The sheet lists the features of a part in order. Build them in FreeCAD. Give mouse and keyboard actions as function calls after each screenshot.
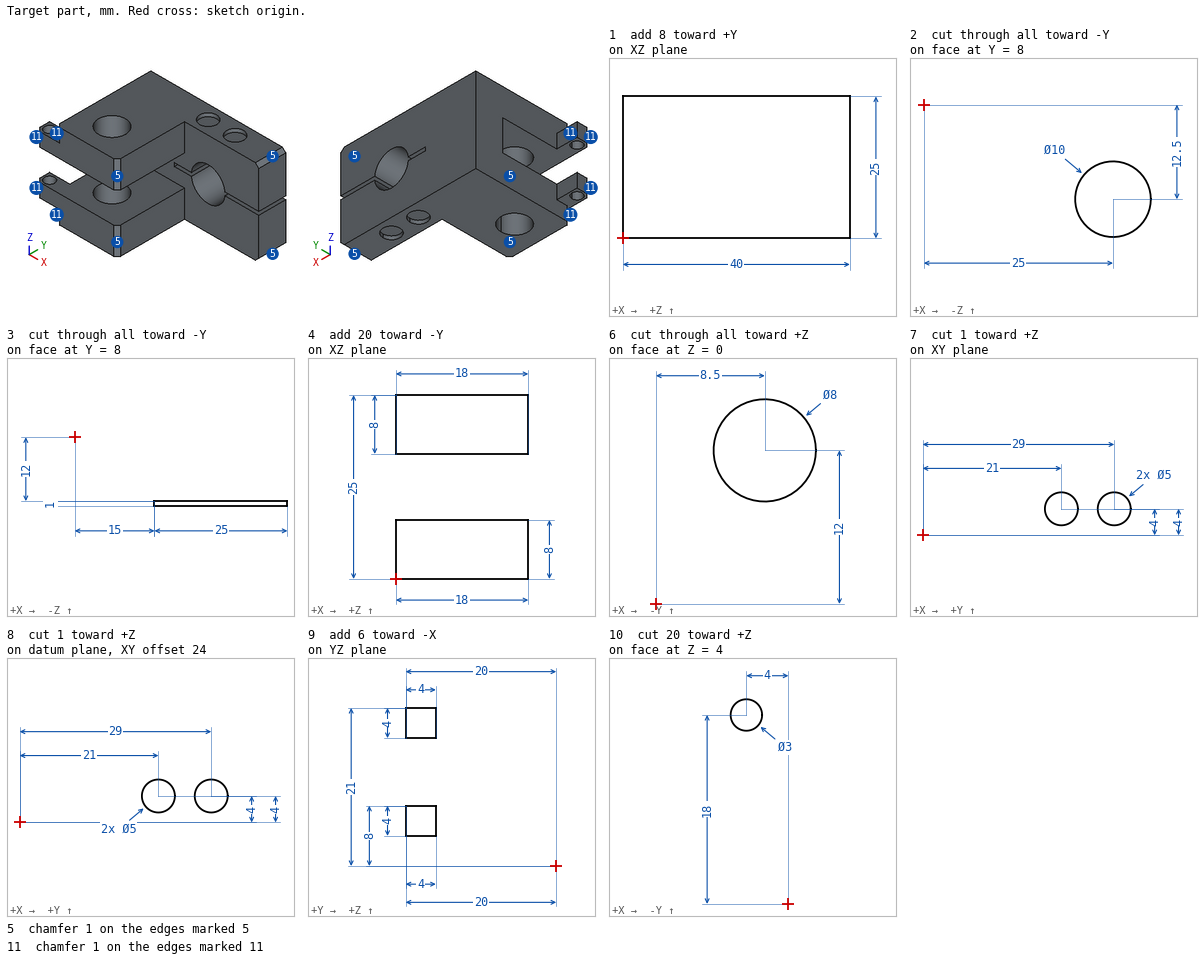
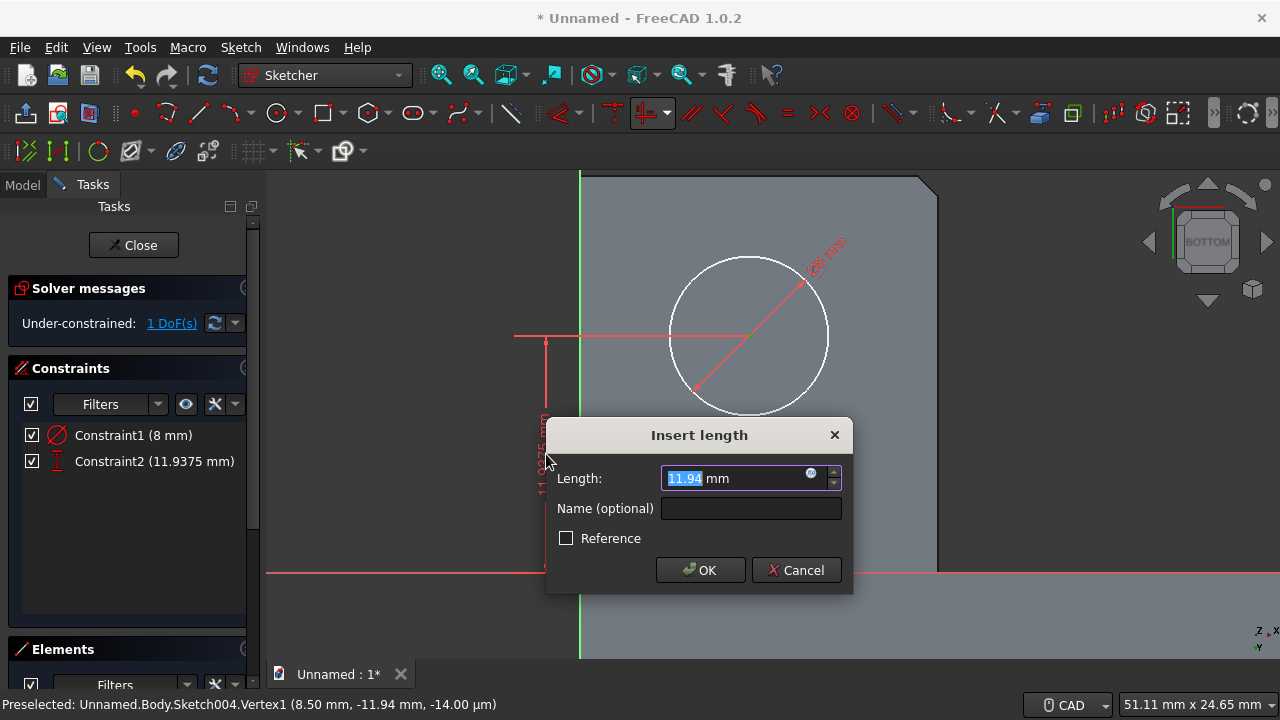
text(12)
key(Return)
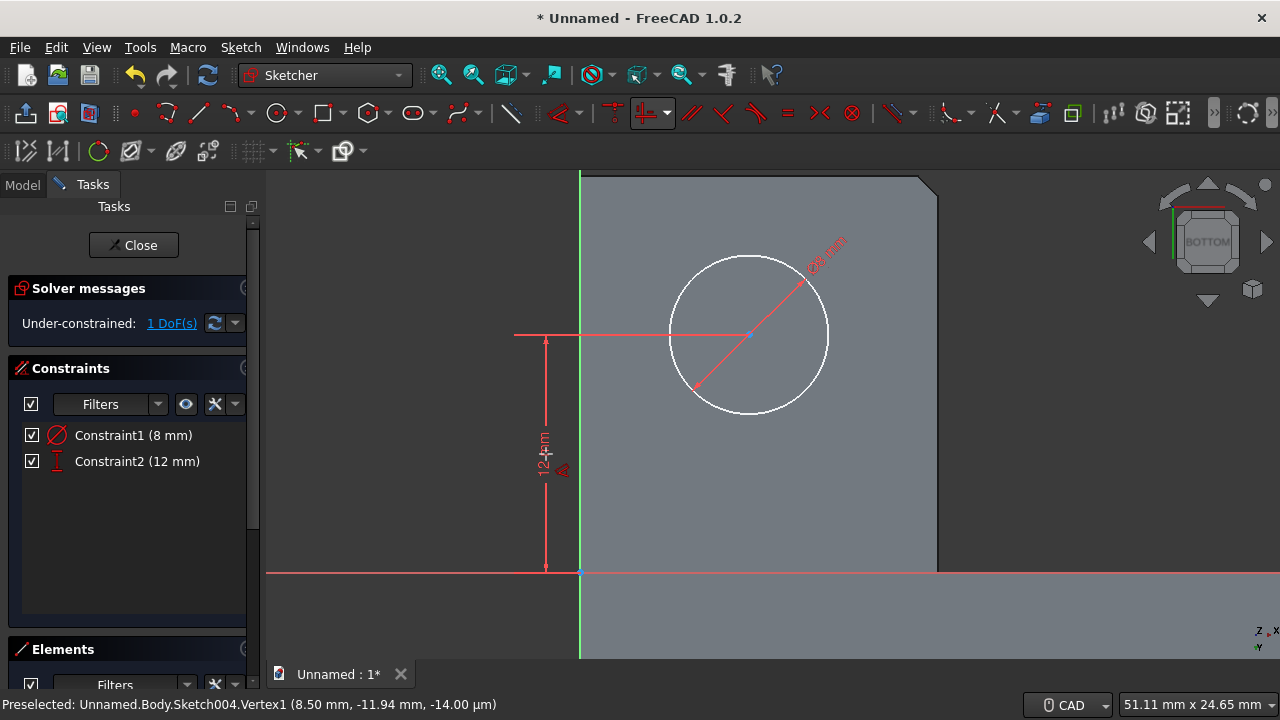
click(749, 335)
click(665, 607)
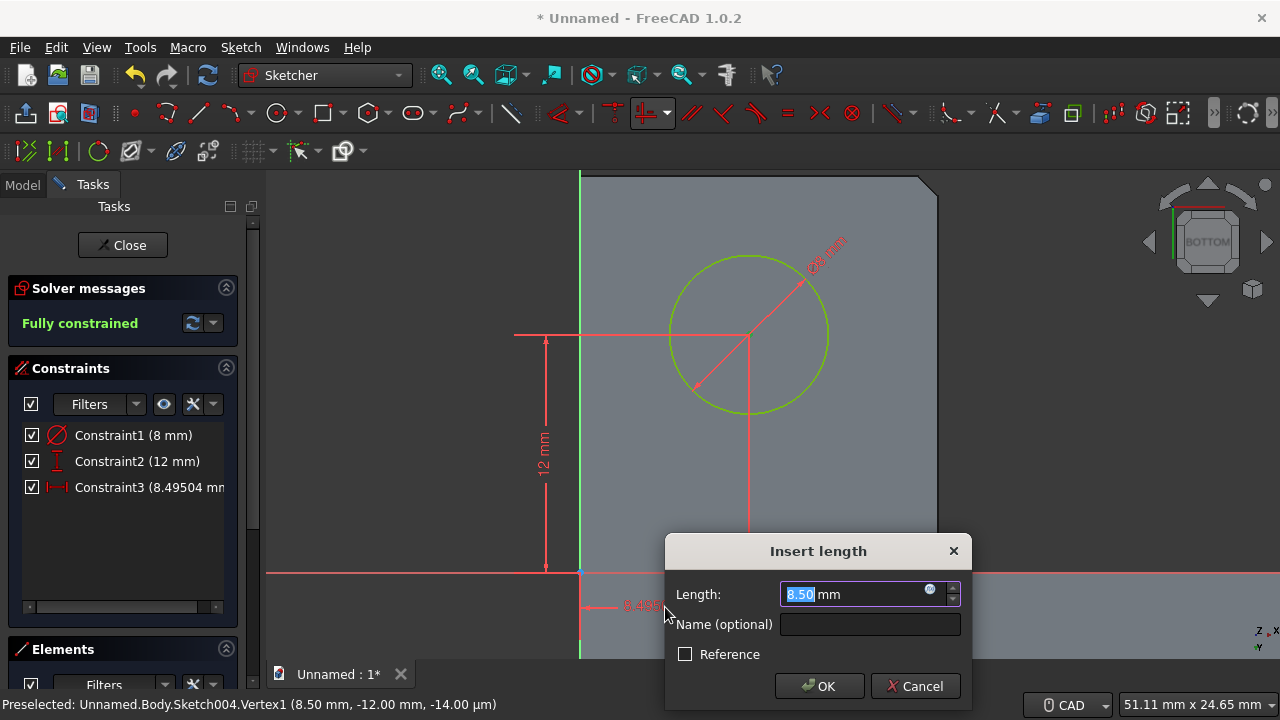
text(8.5)
key(Return)
key(Escape)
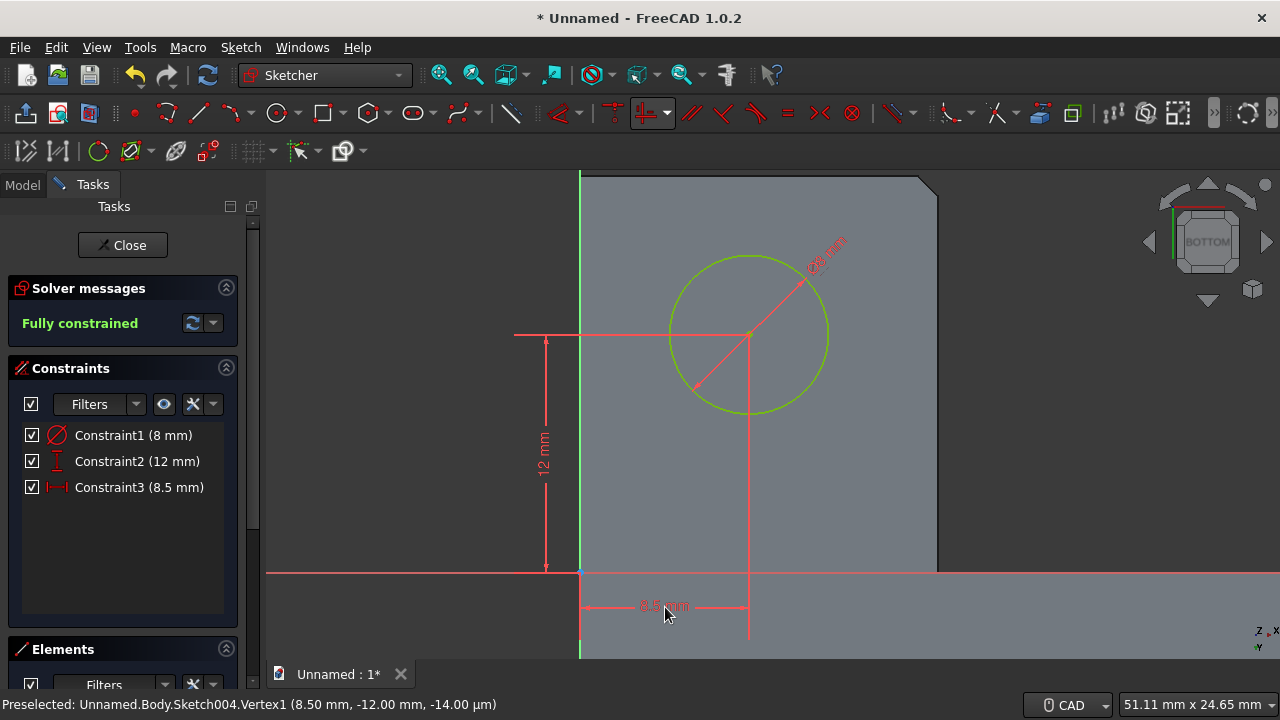
click(123, 245)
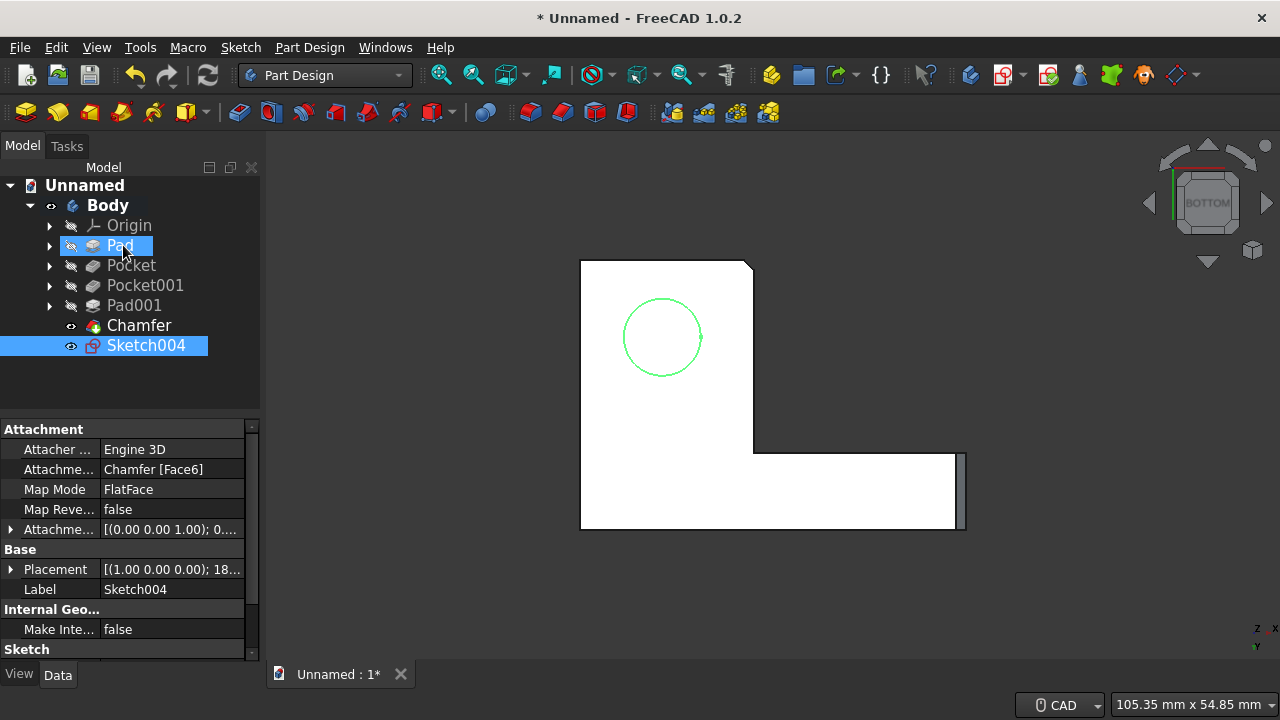
click(240, 112)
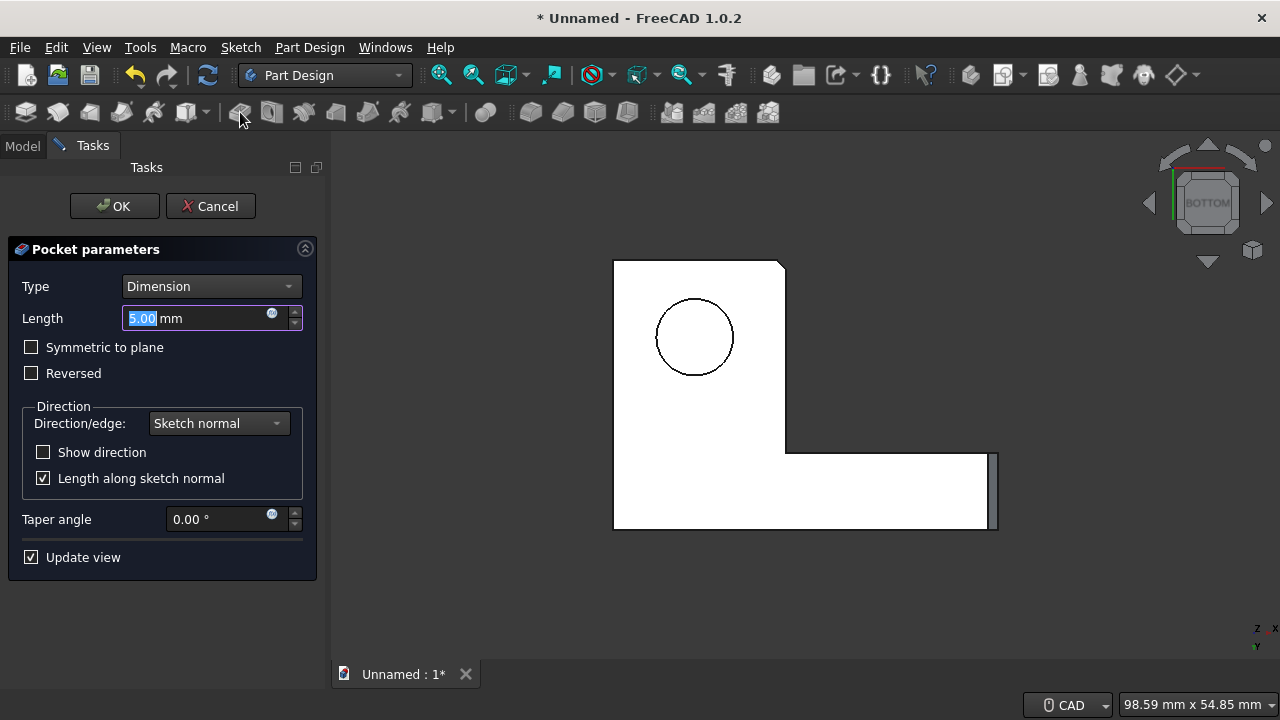
click(212, 286)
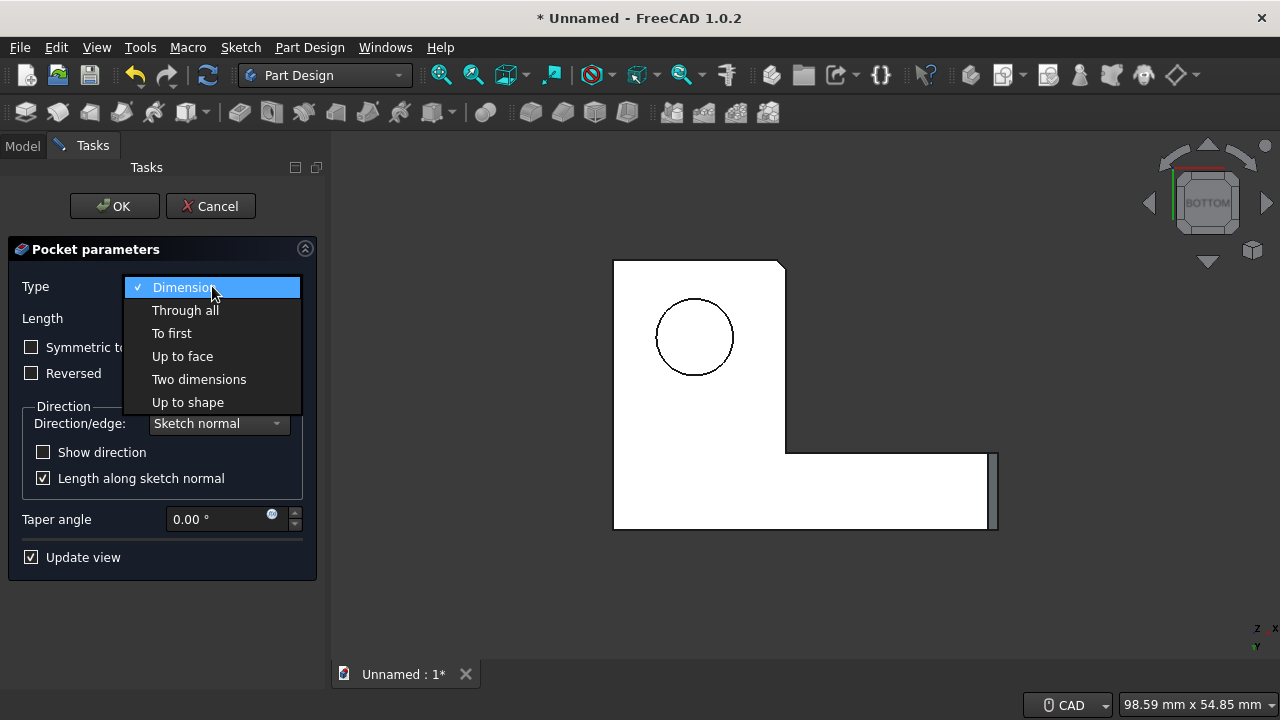
click(212, 310)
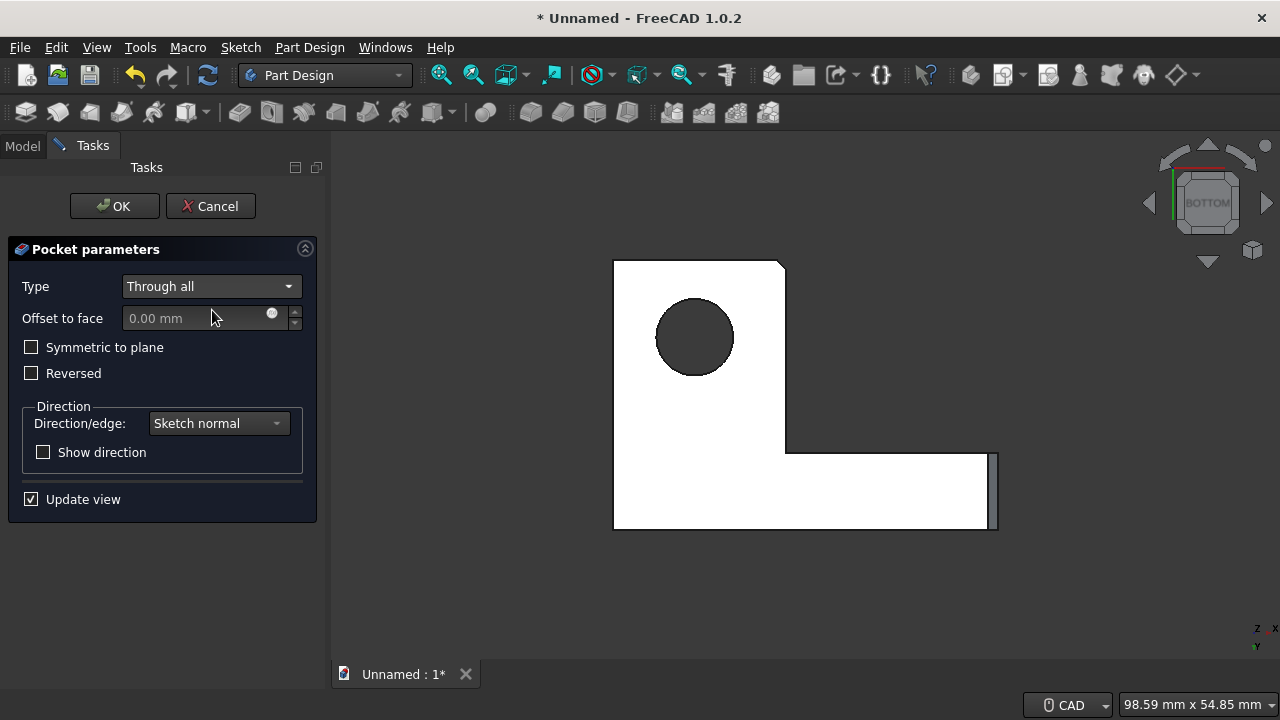
click(115, 206)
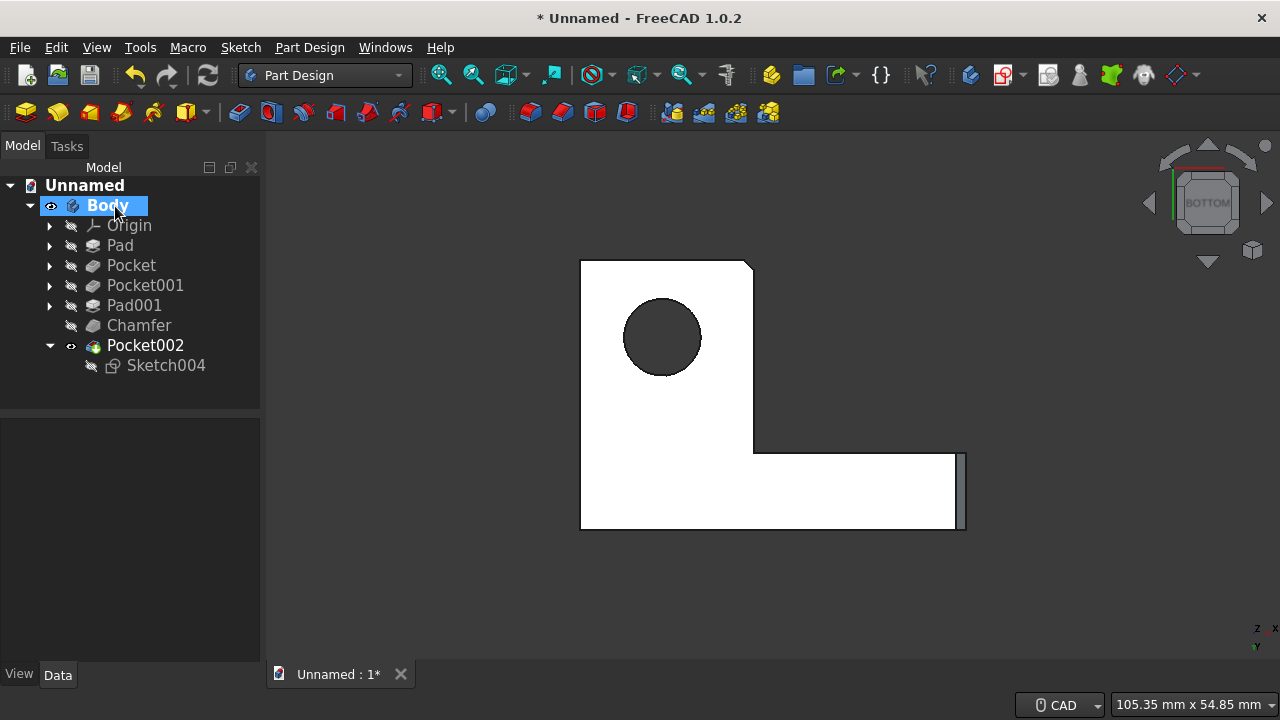
click(1004, 76)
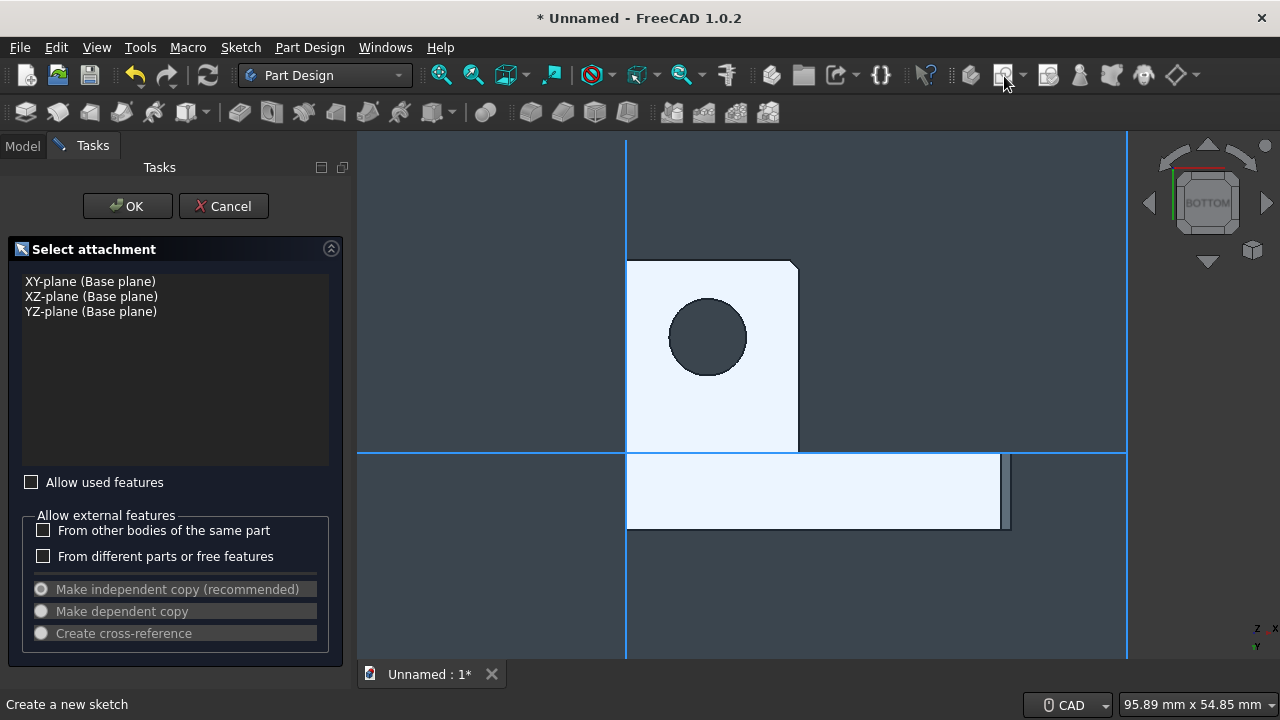
click(82, 282)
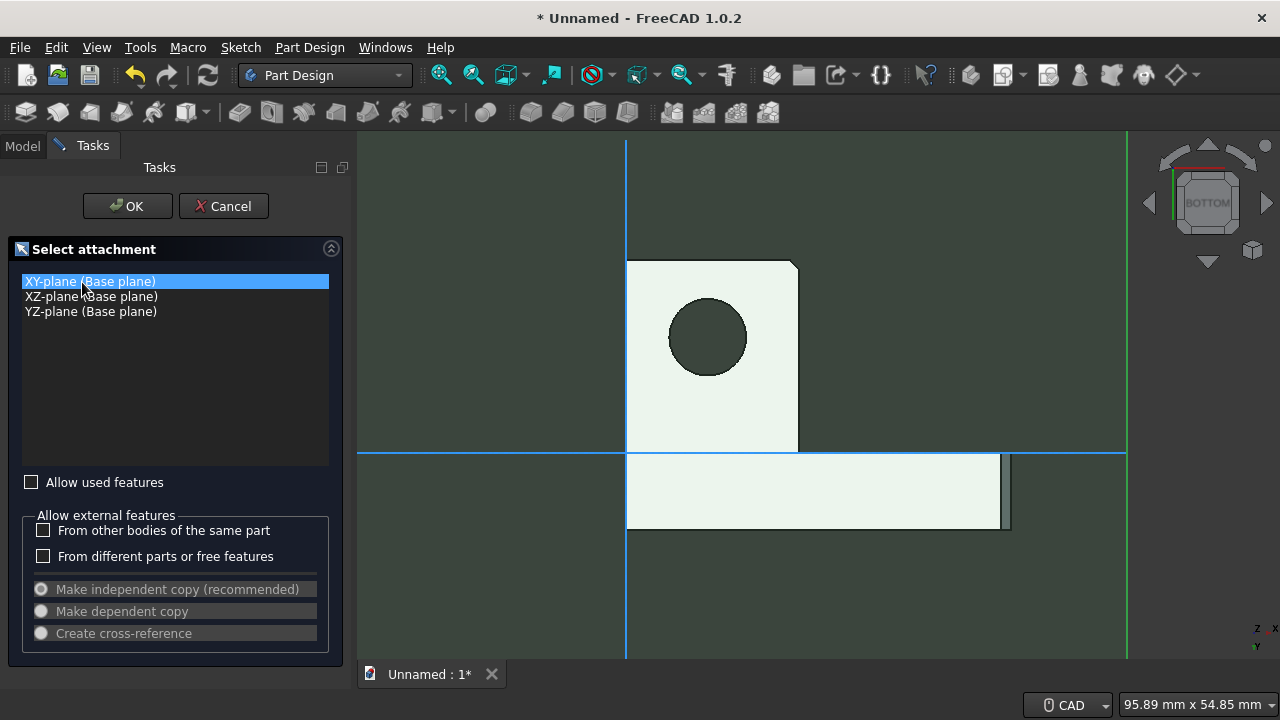
click(128, 206)